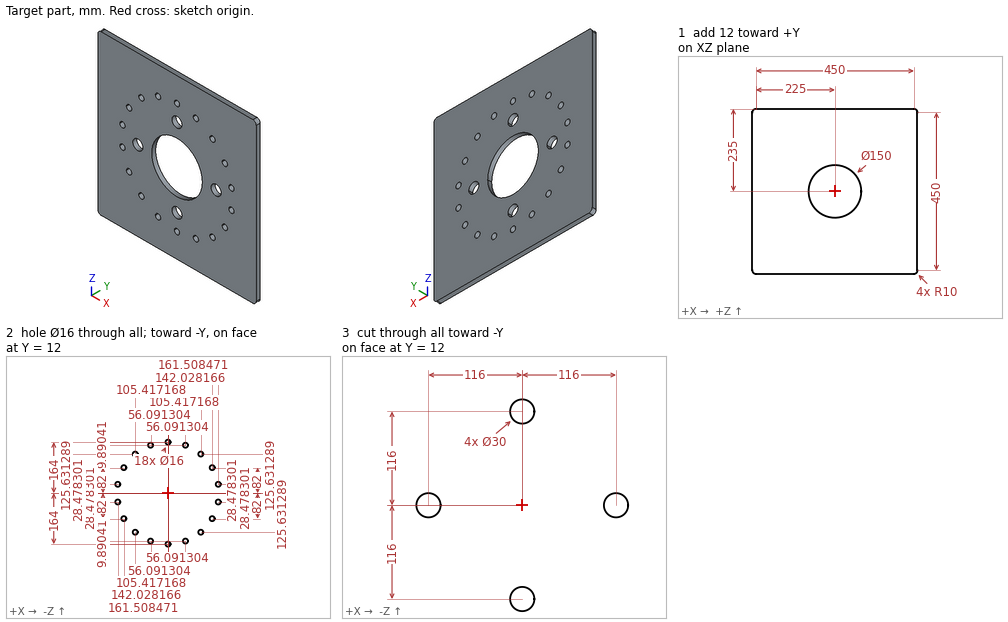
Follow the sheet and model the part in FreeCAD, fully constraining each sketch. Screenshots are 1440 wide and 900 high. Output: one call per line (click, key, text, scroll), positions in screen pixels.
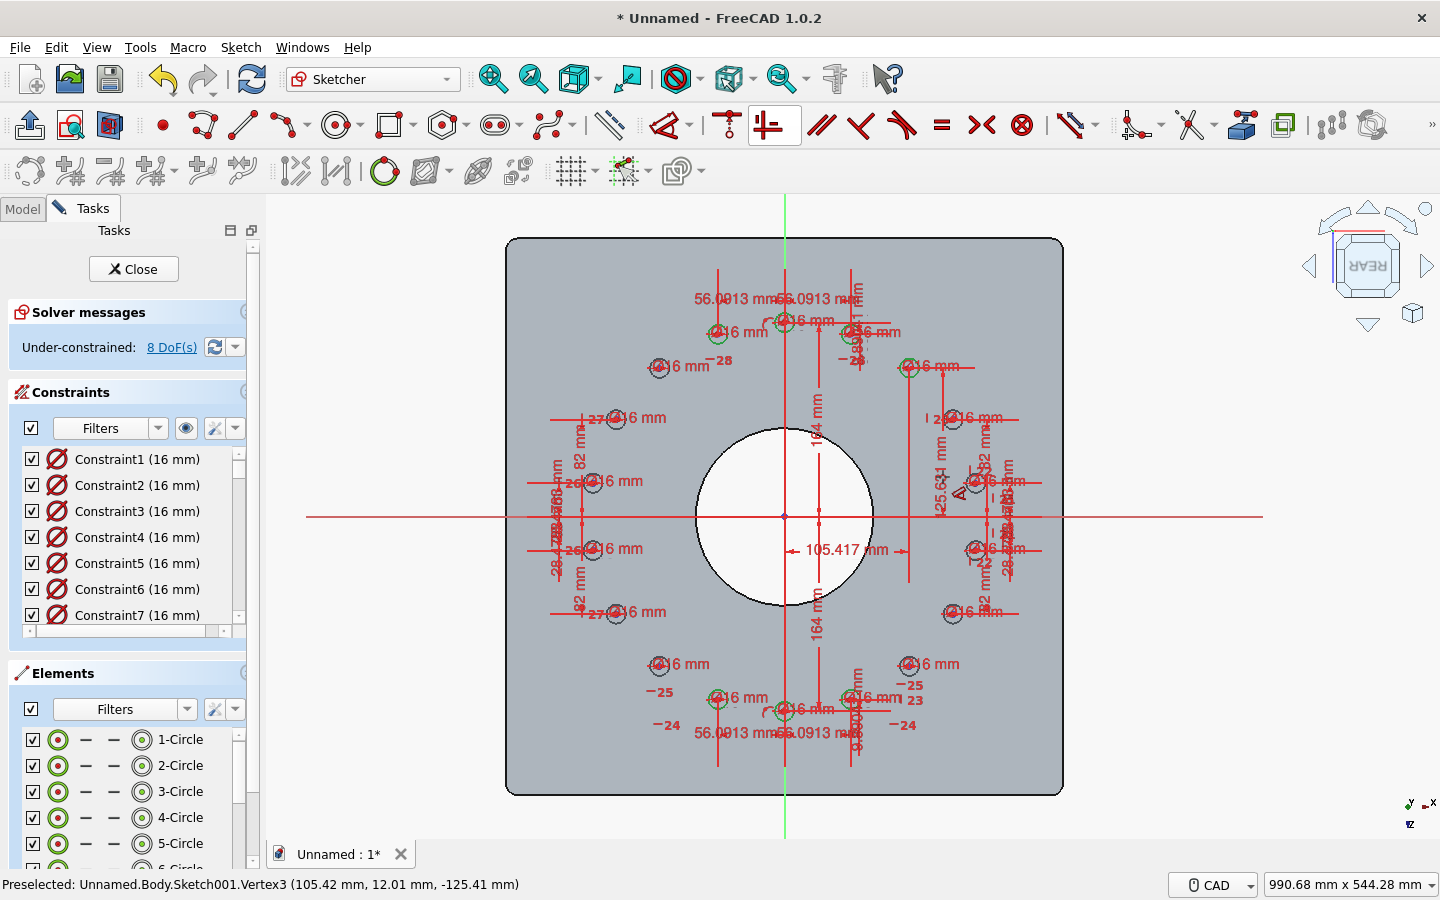
click(953, 420)
click(869, 386)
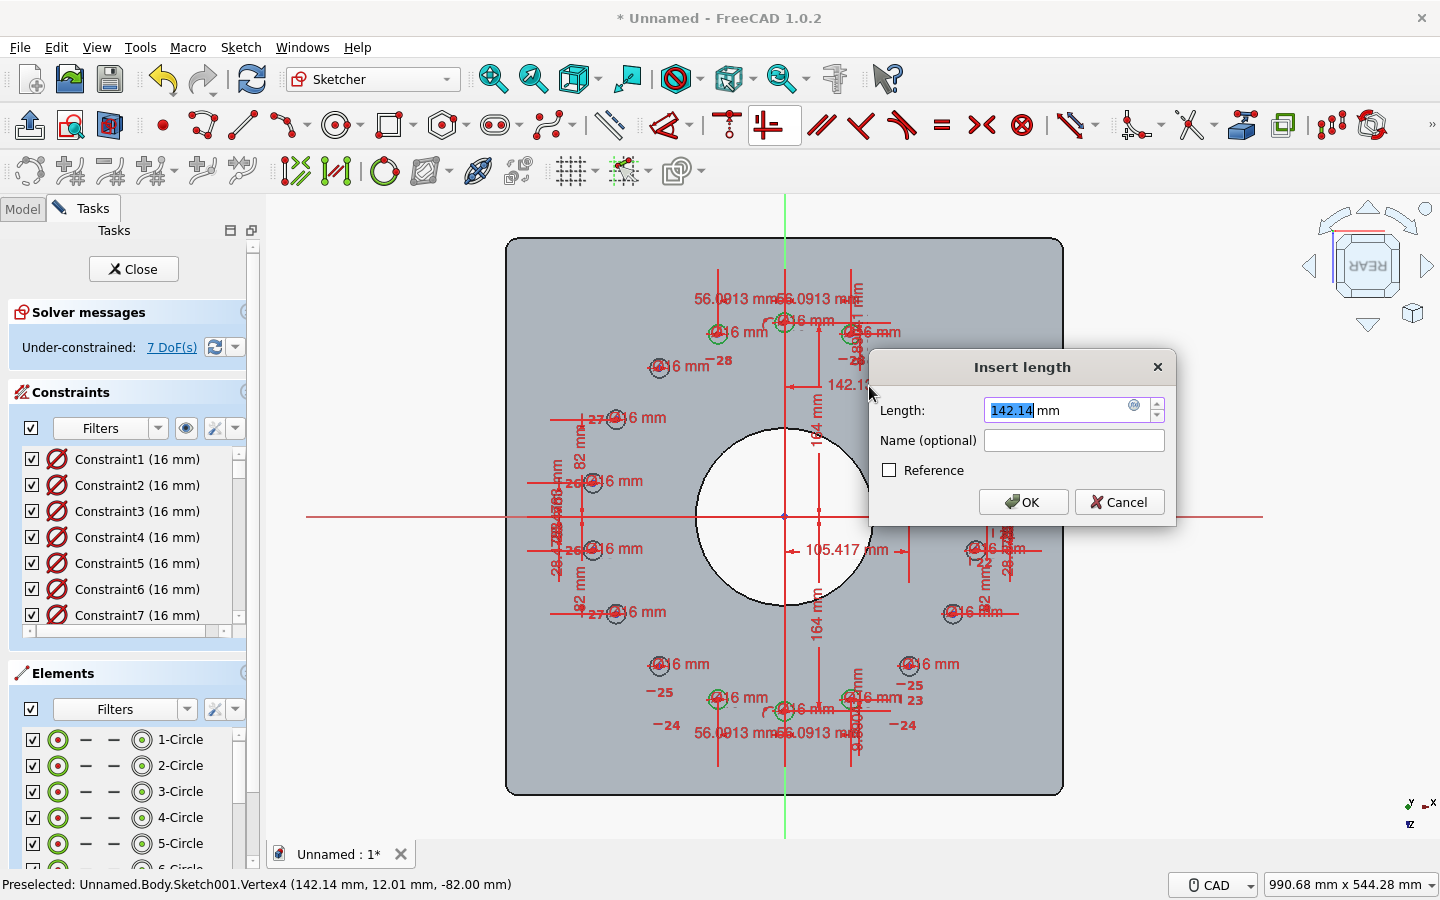
text(142.028166)
key(Return)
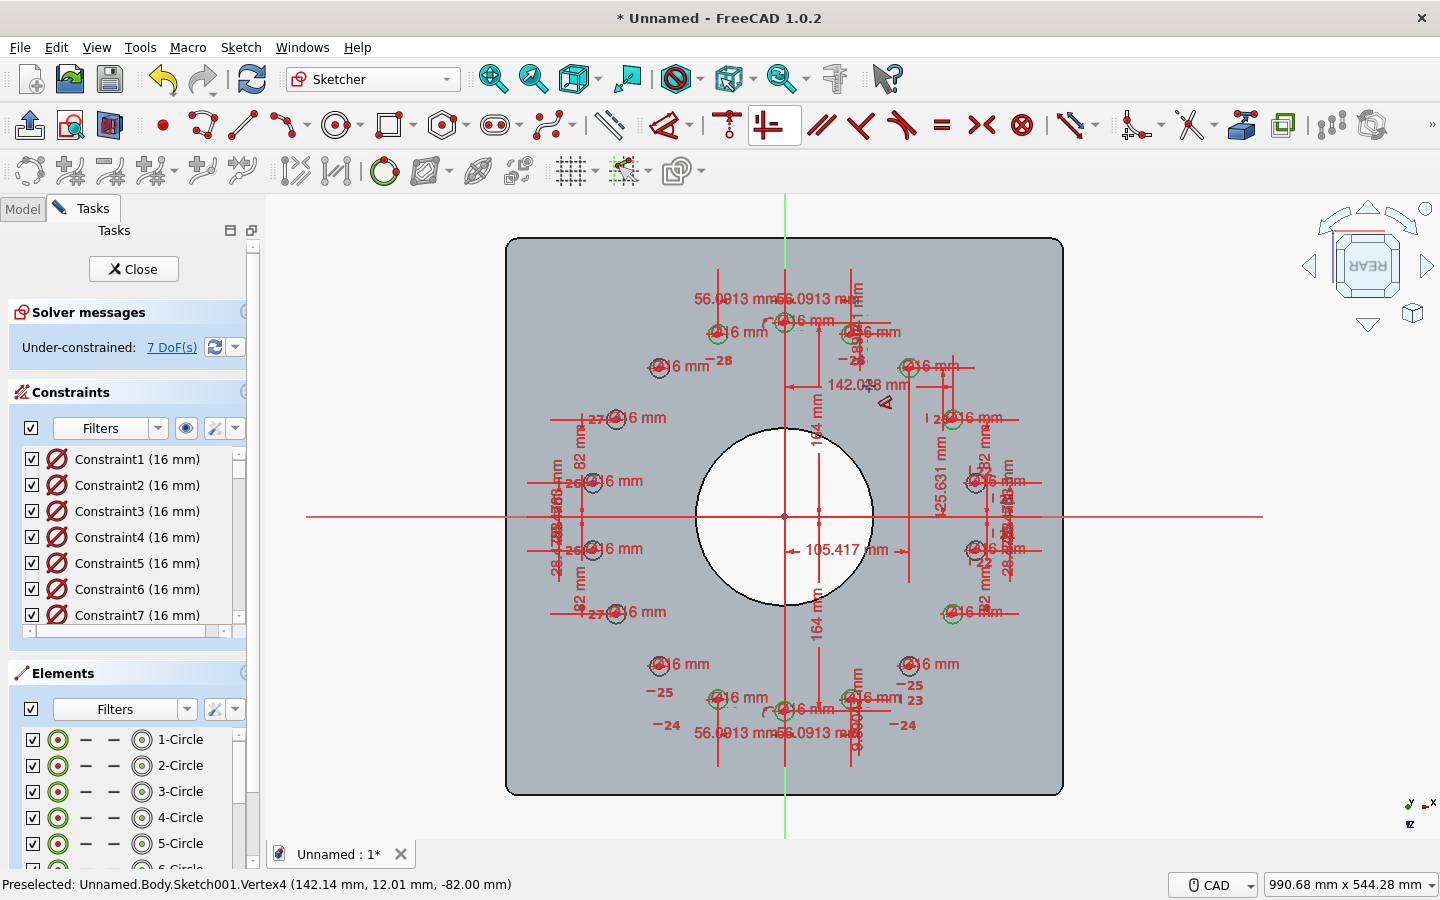
click(976, 483)
click(880, 449)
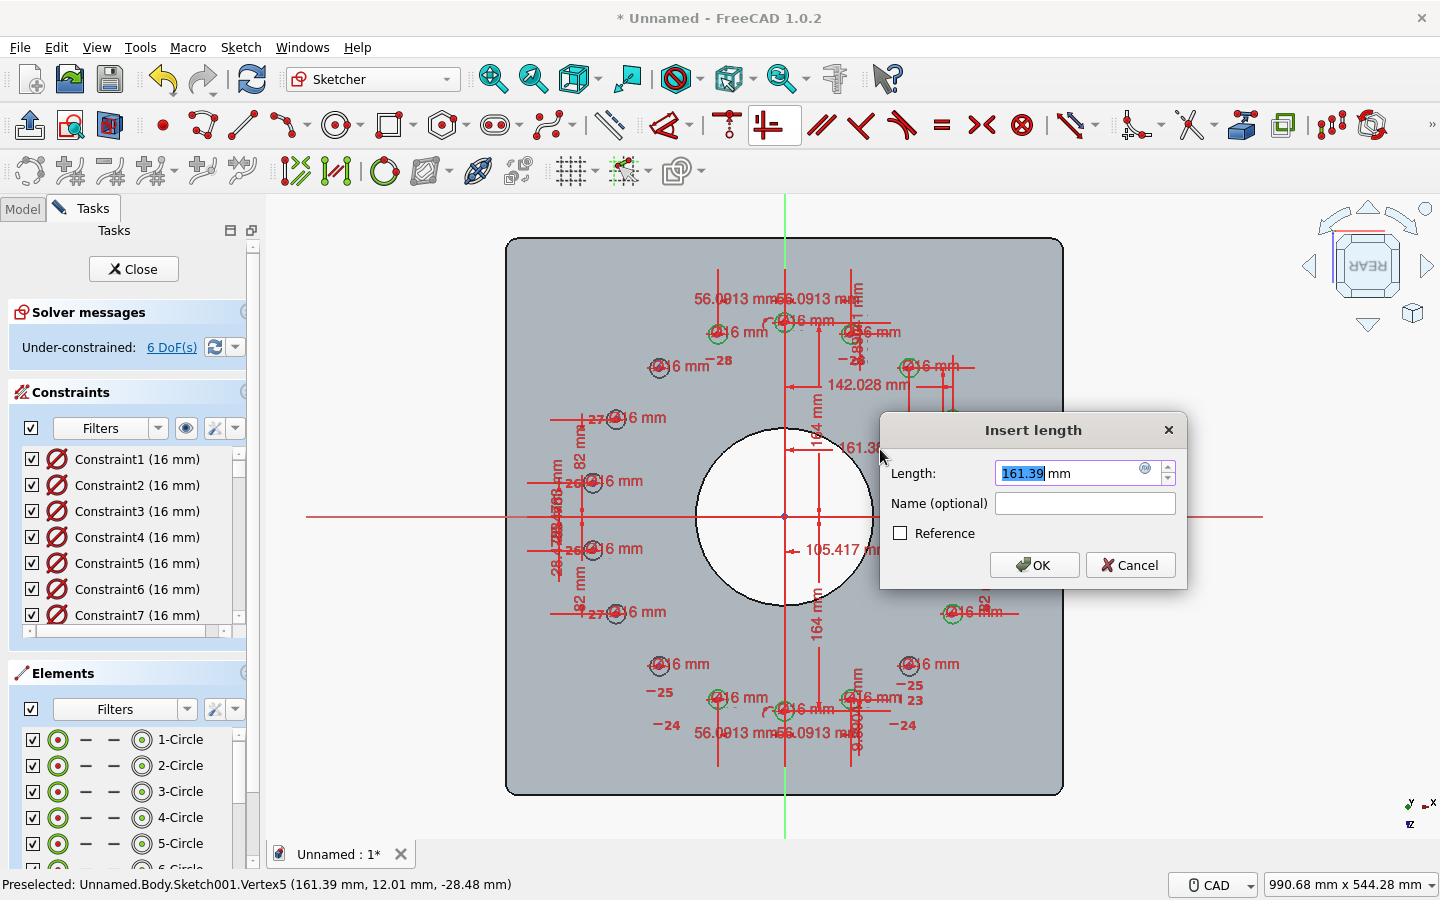
text(161.508471)
key(Return)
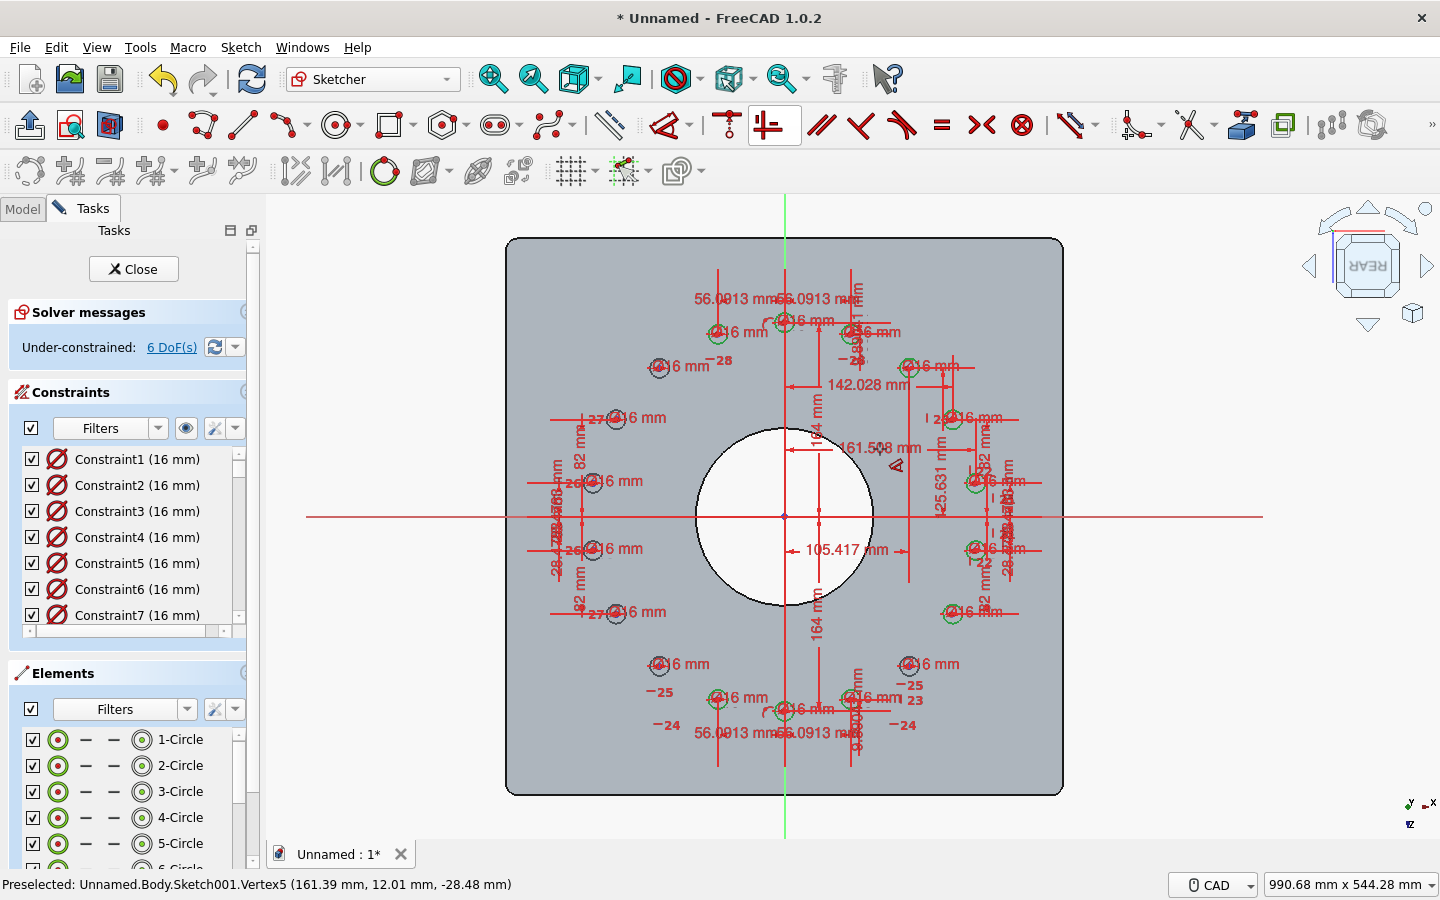
click(909, 666)
click(943, 557)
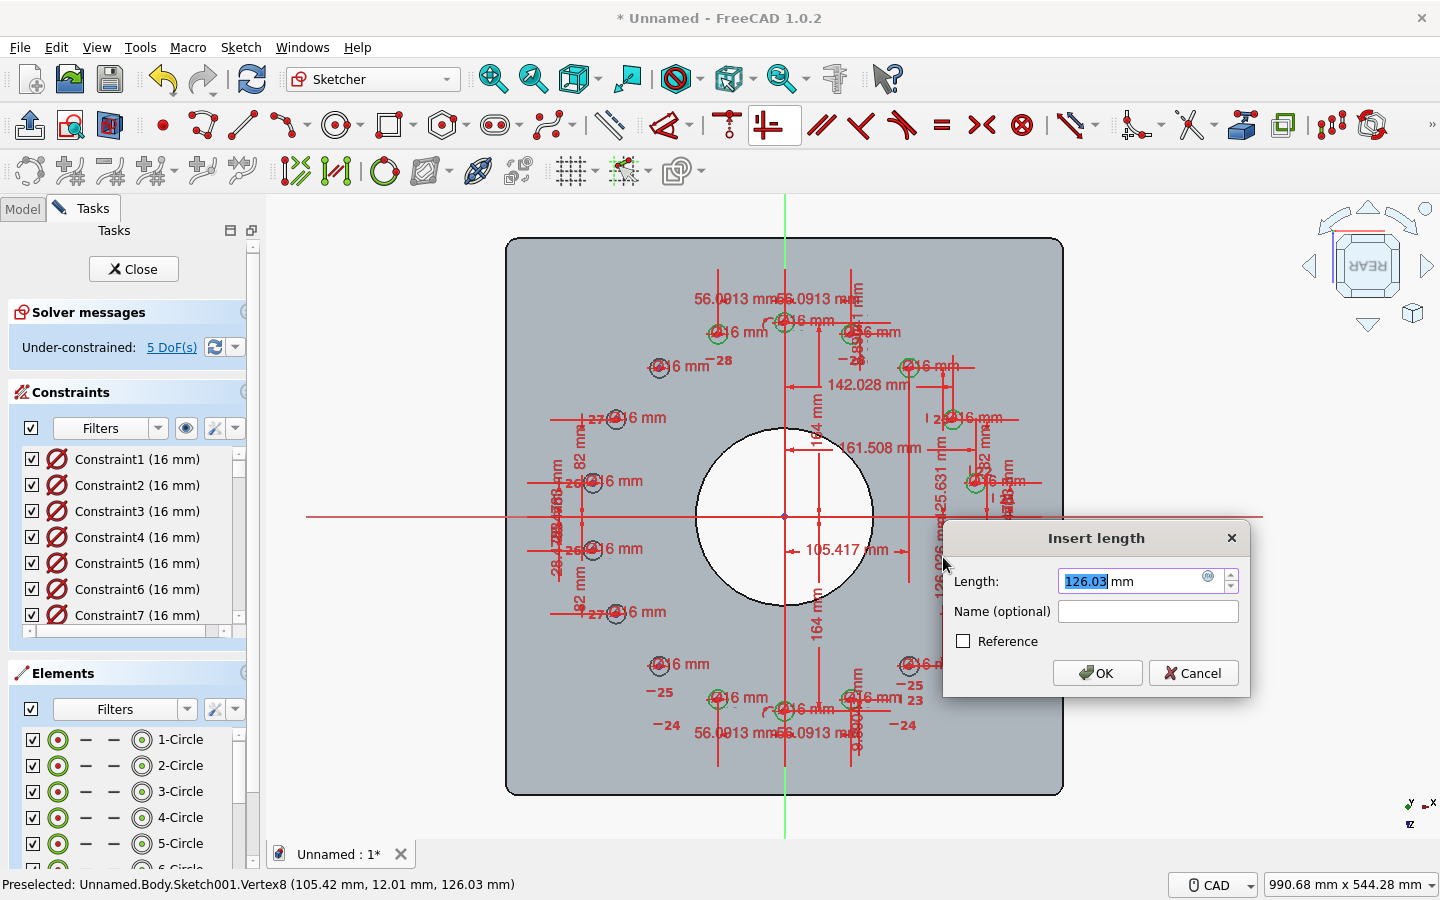
text(125.631289)
key(Return)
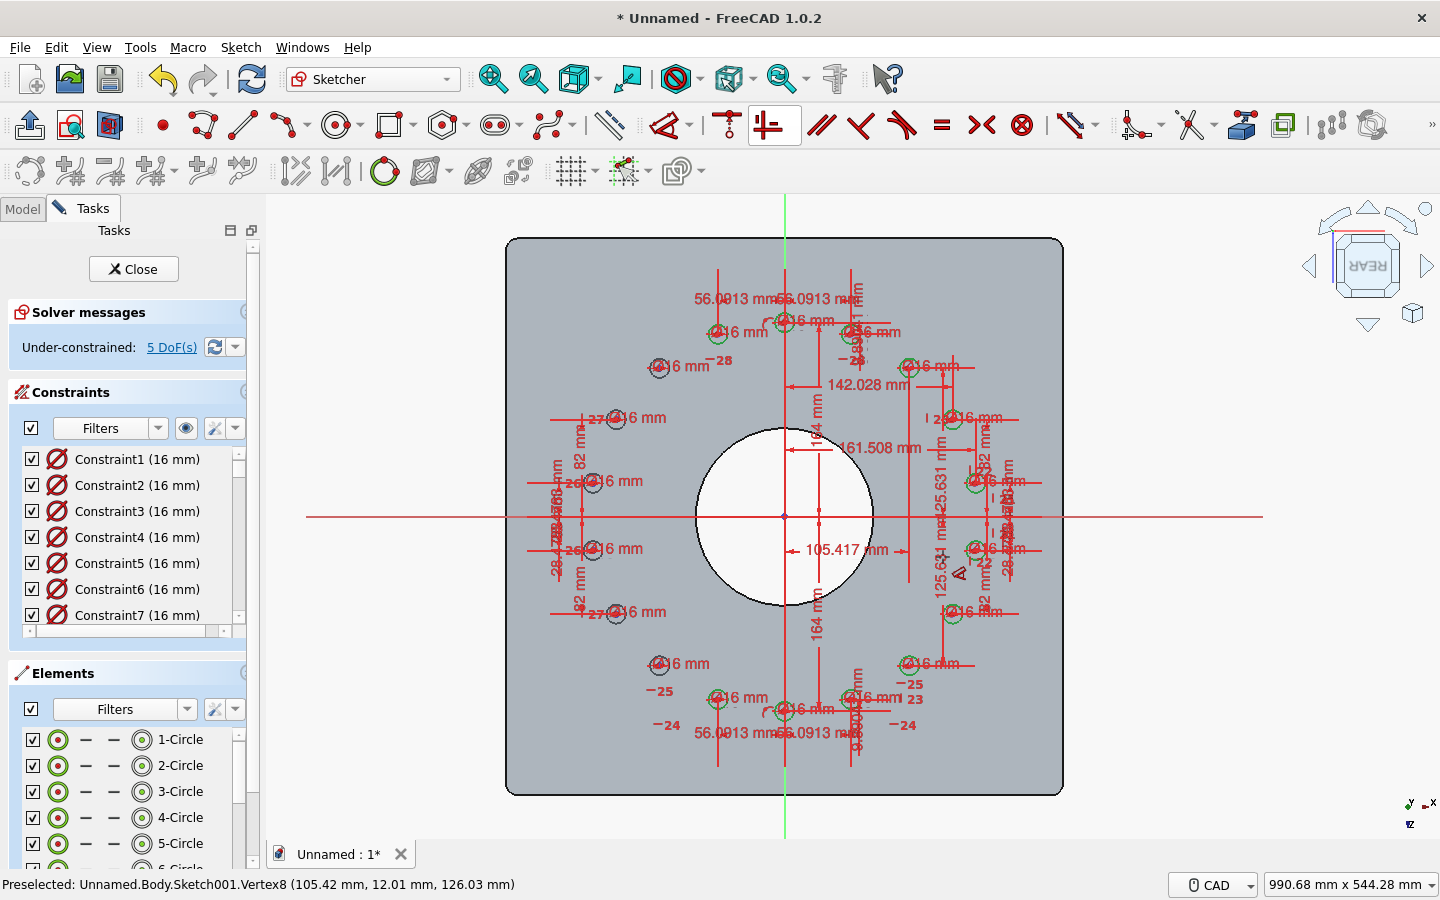
click(660, 666)
click(693, 700)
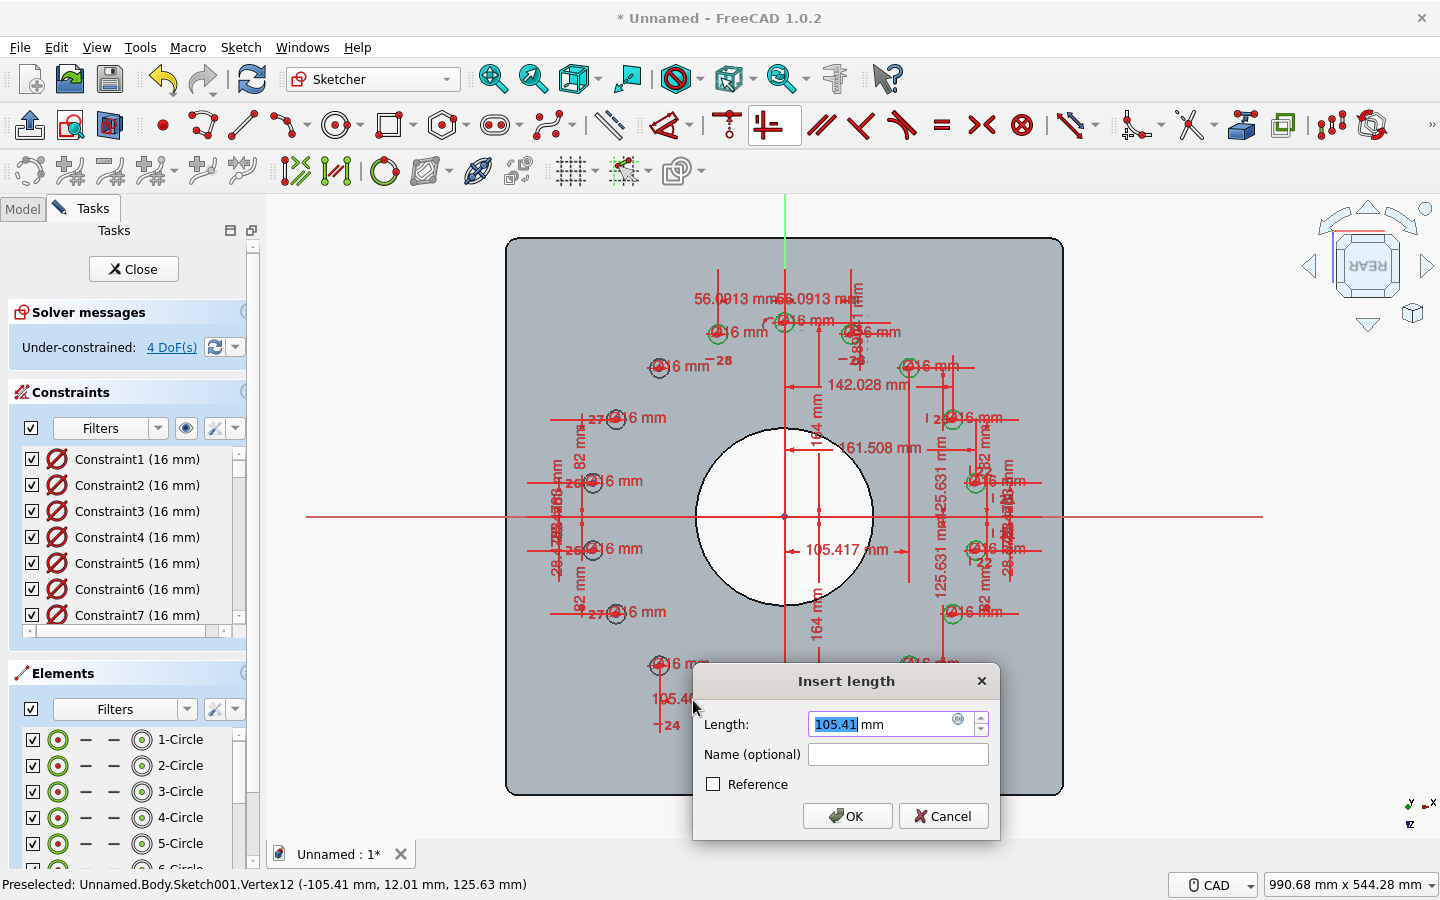
text(105.417168)
key(Return)